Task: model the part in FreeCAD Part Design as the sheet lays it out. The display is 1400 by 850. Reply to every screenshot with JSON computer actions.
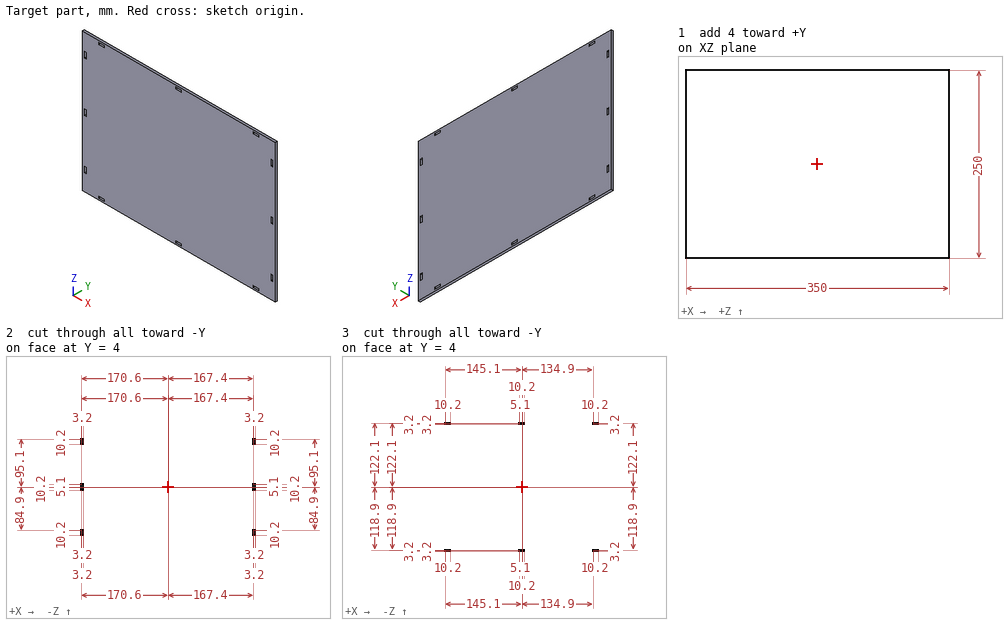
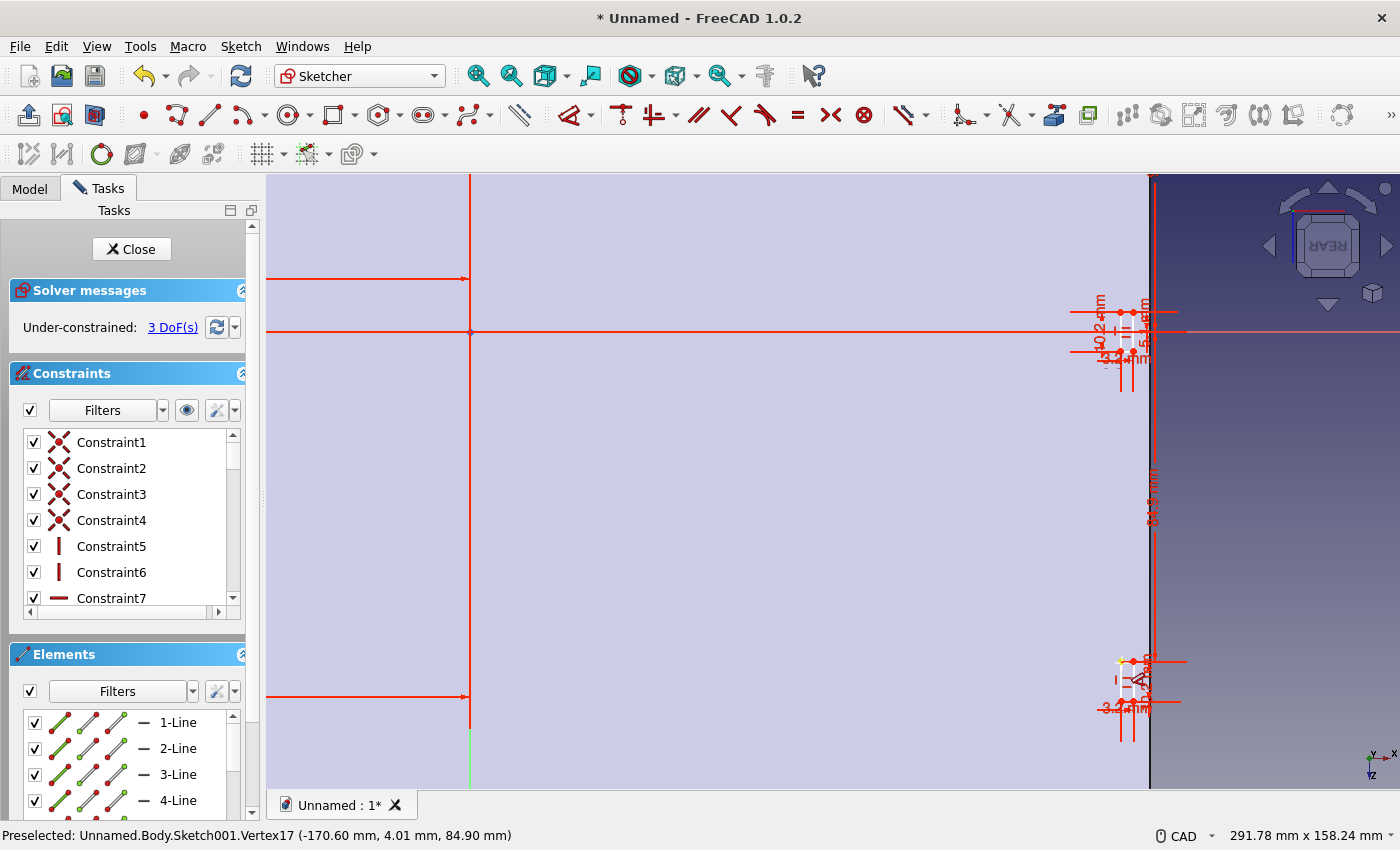
{"action": "left_click", "coordinate": [1121, 662]}
{"action": "left_click", "coordinate": [796, 696]}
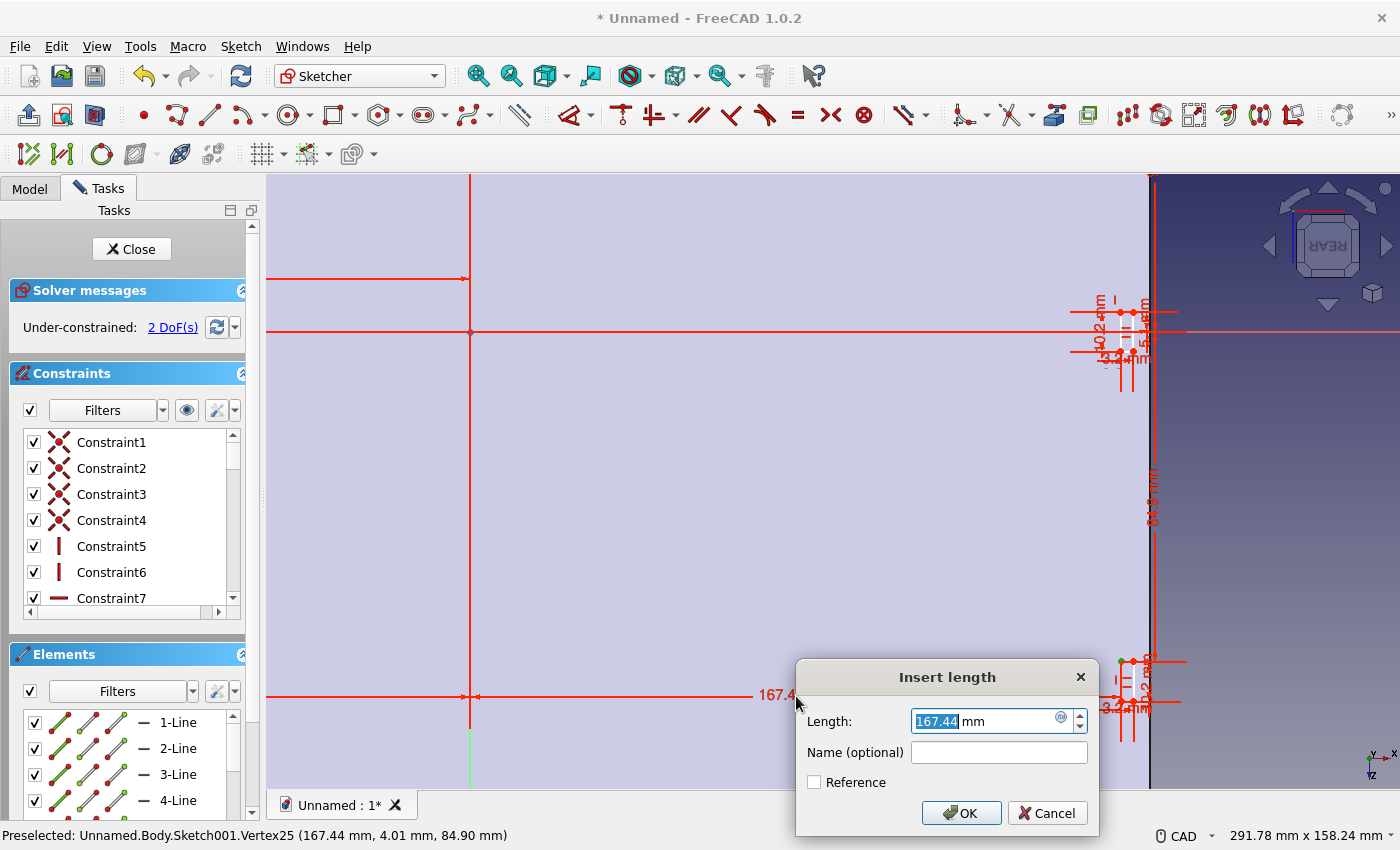
{"action": "type", "text": "167.4"}
{"action": "key", "text": "Return"}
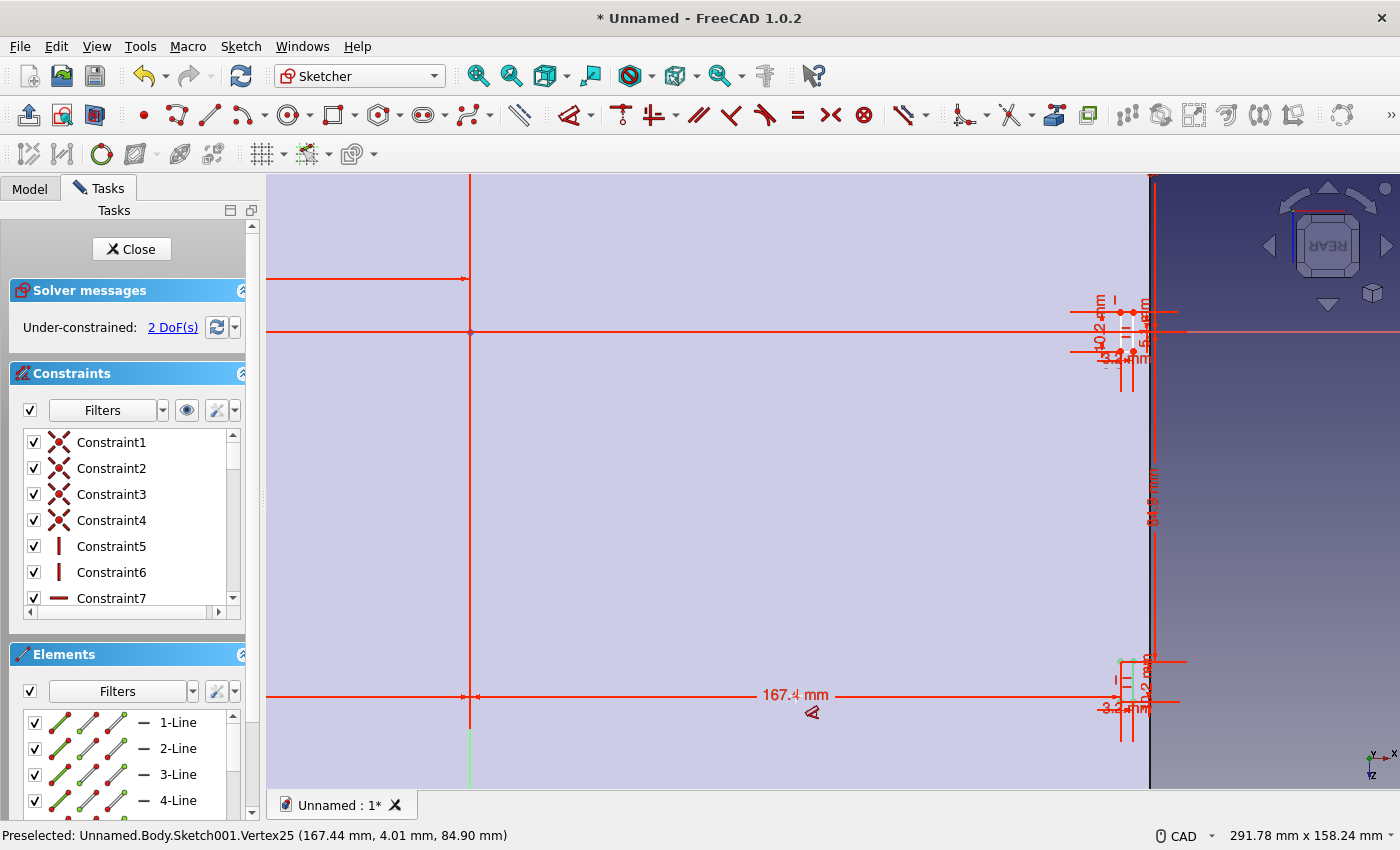
{"action": "left_click", "coordinate": [1121, 312]}
{"action": "left_click", "coordinate": [796, 278]}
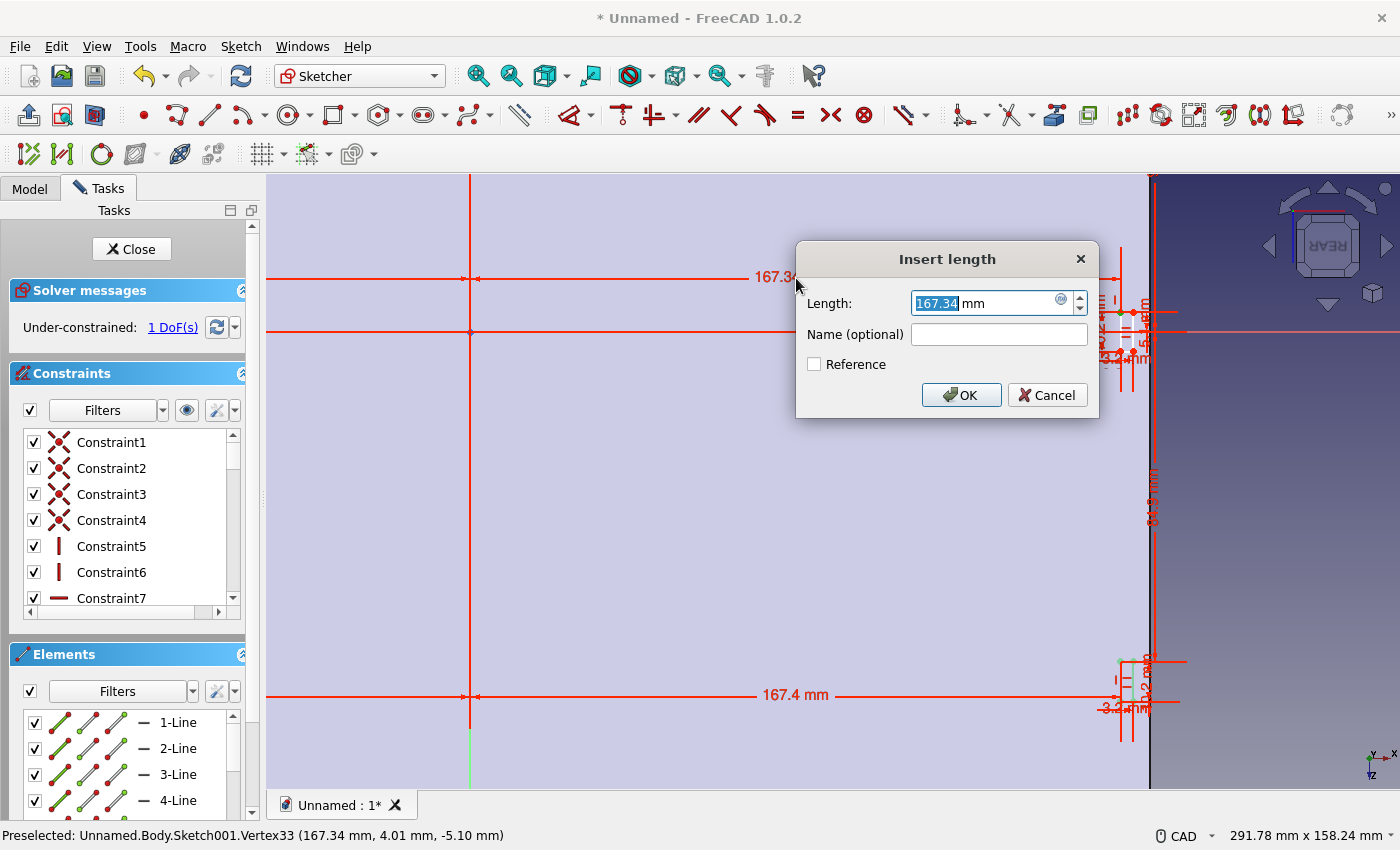
{"action": "type", "text": "167.4"}
{"action": "key", "text": "Return"}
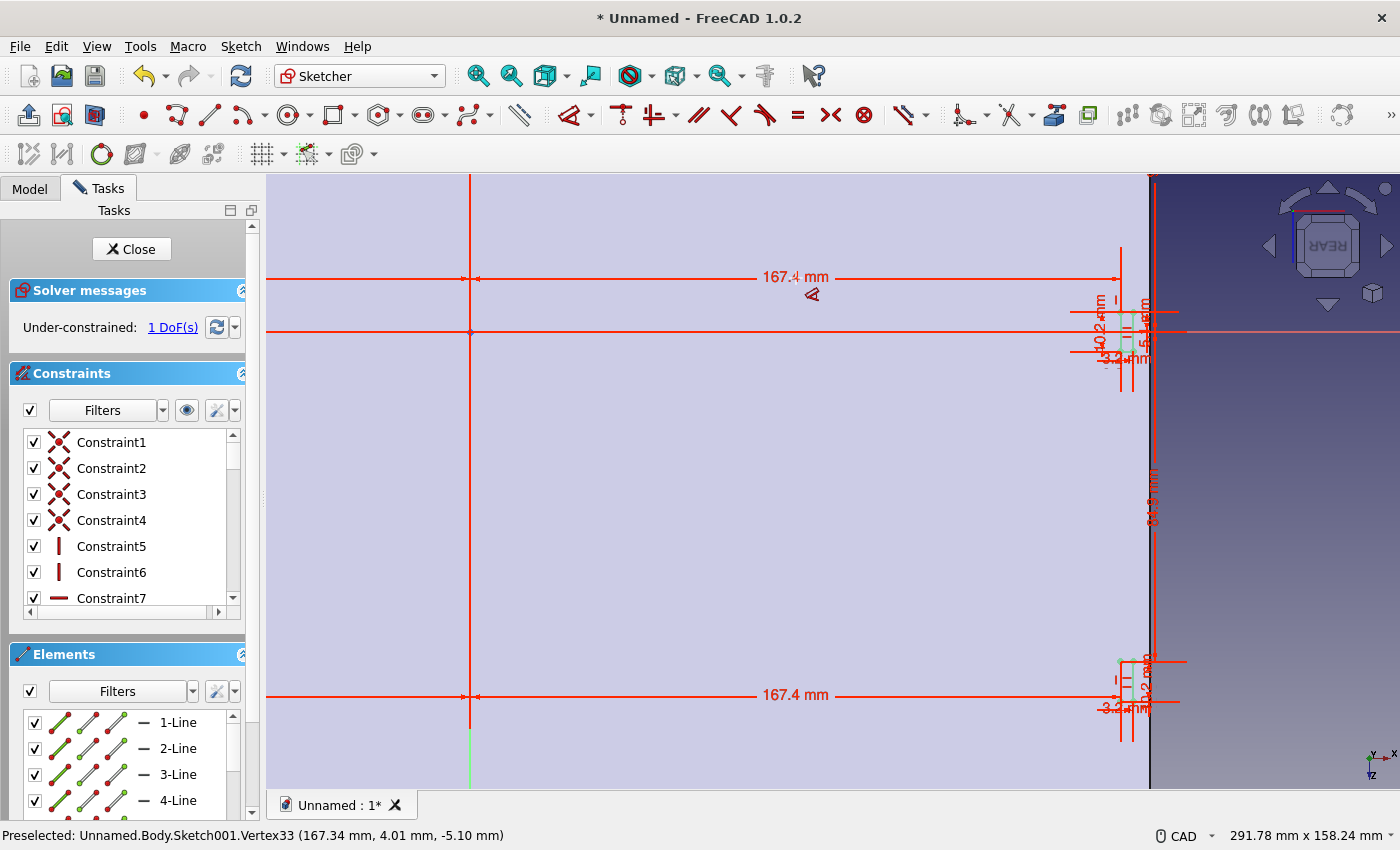
{"action": "scroll", "coordinate": [1122, 663], "scroll_direction": "down", "scroll_amount": 3}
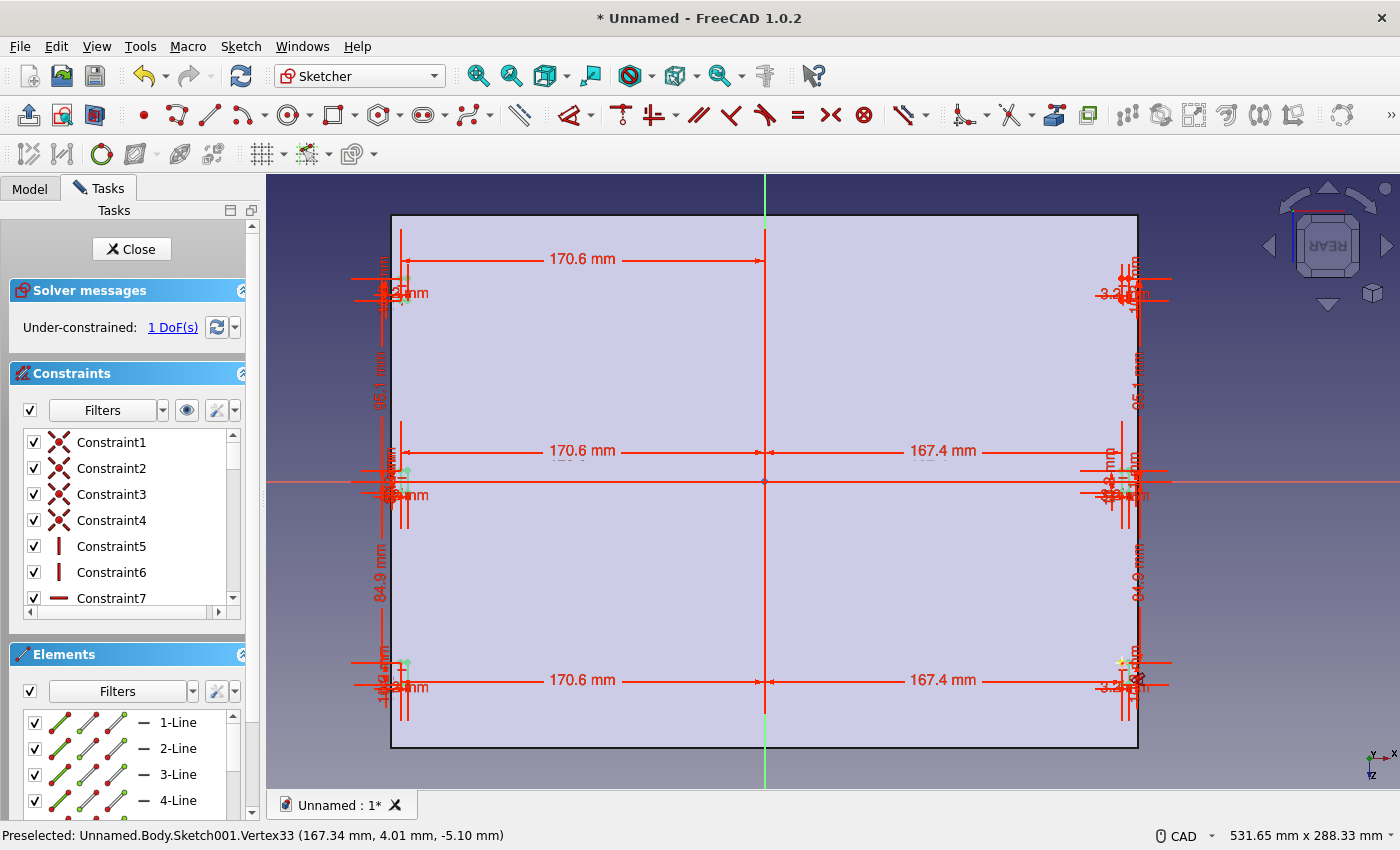
{"action": "scroll", "coordinate": [1122, 279], "scroll_direction": "up", "scroll_amount": 3}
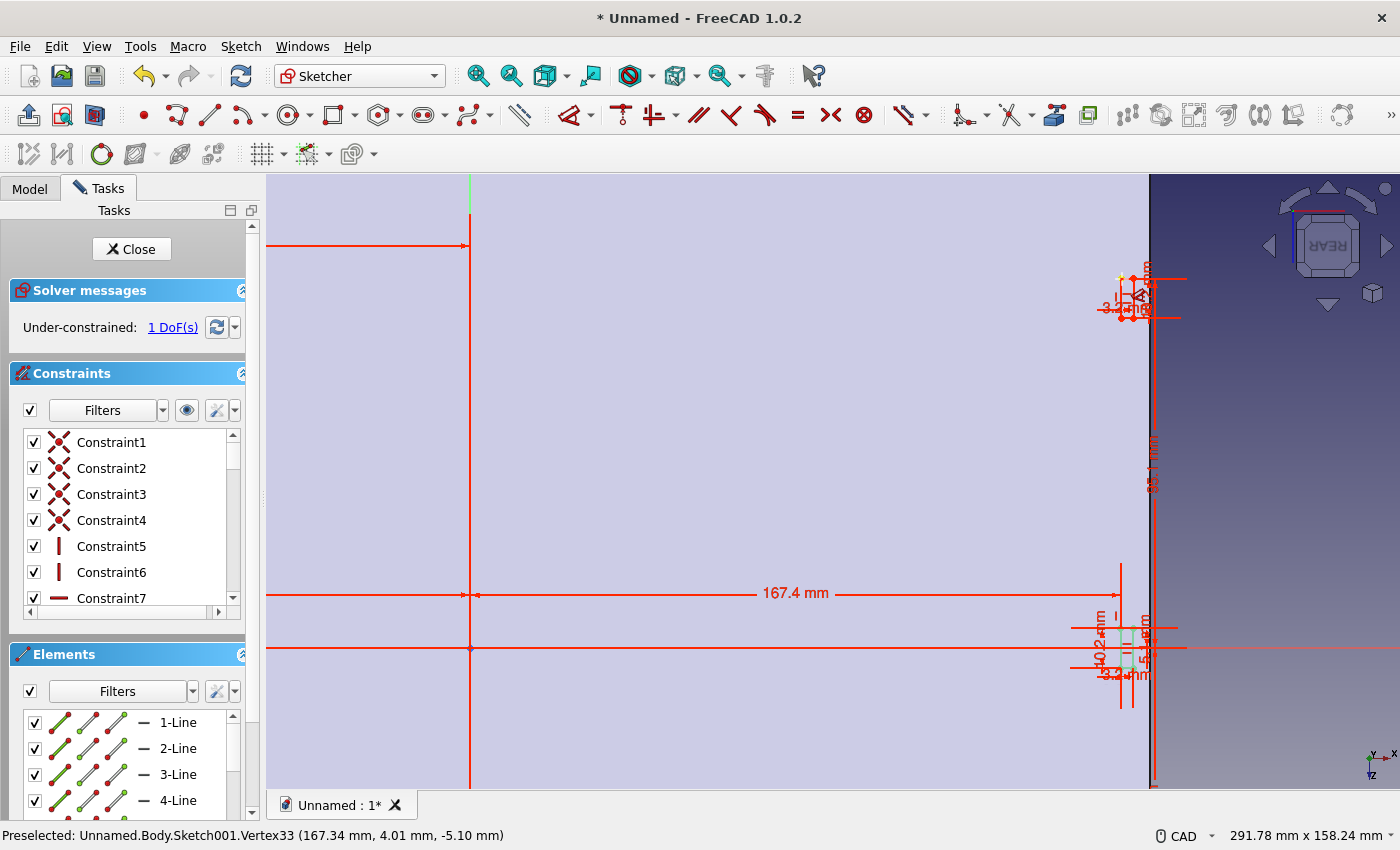
{"action": "left_click", "coordinate": [1121, 279]}
{"action": "left_click", "coordinate": [796, 245]}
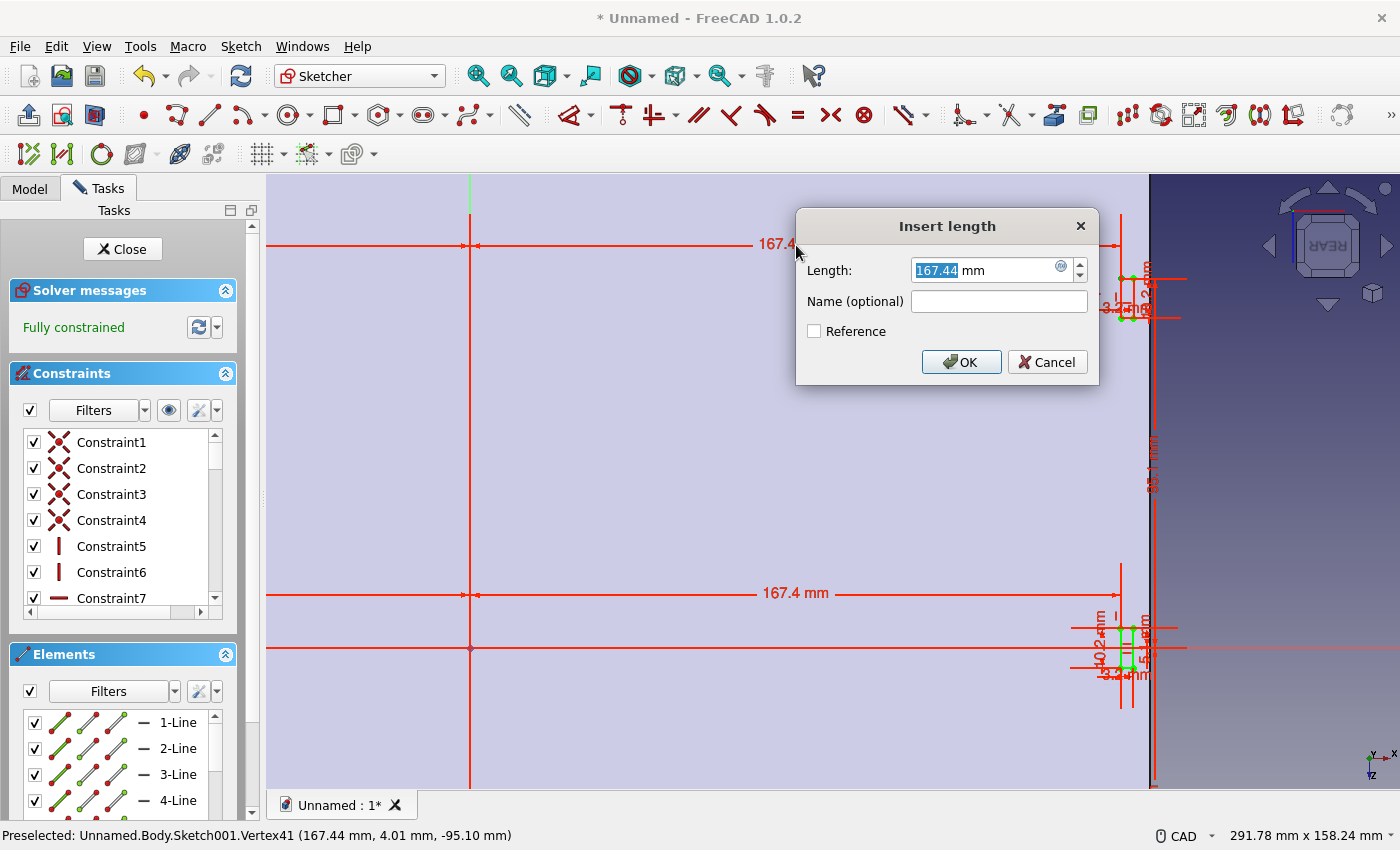
{"action": "type", "text": "167.4"}
{"action": "key", "text": "Return"}
{"action": "key", "text": "Escape"}